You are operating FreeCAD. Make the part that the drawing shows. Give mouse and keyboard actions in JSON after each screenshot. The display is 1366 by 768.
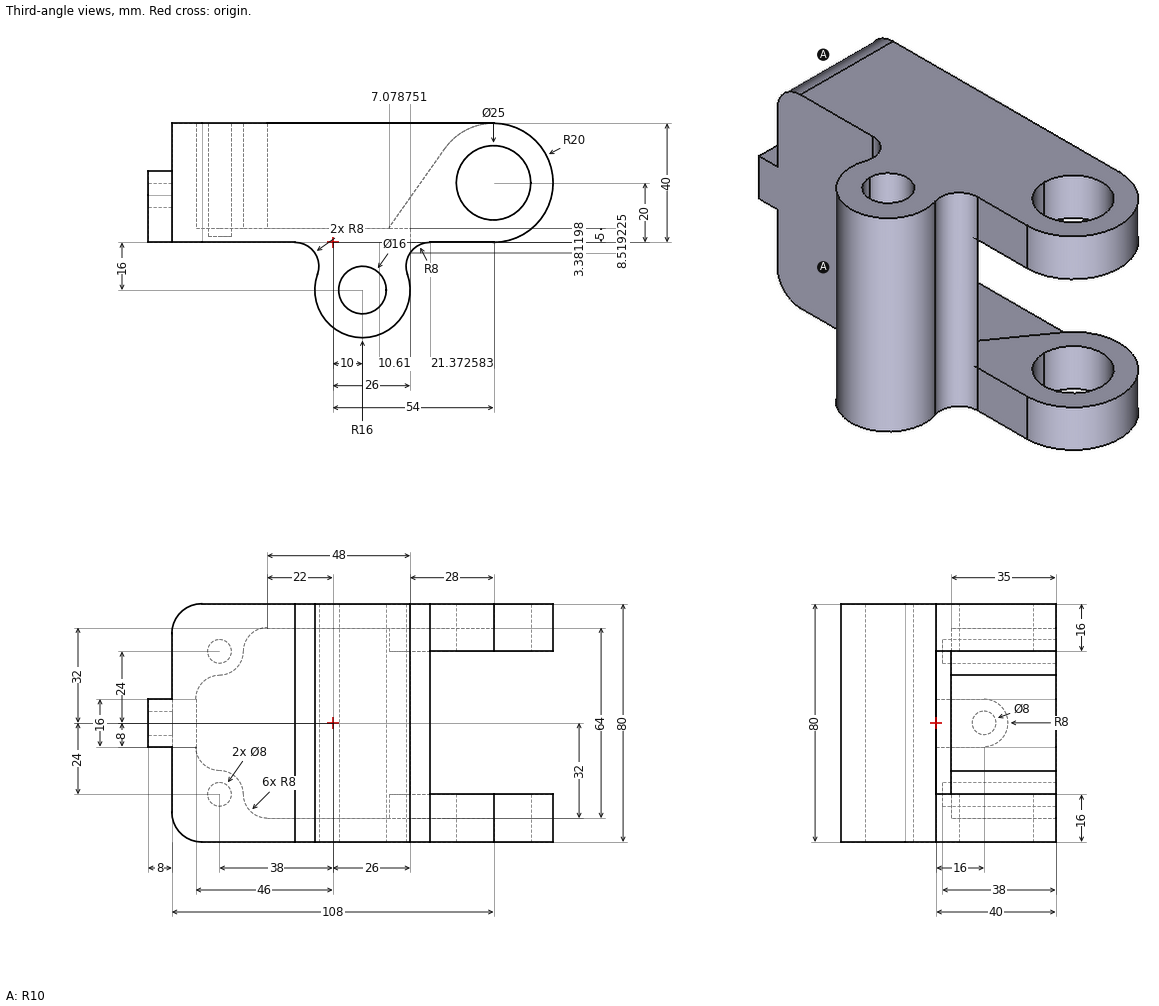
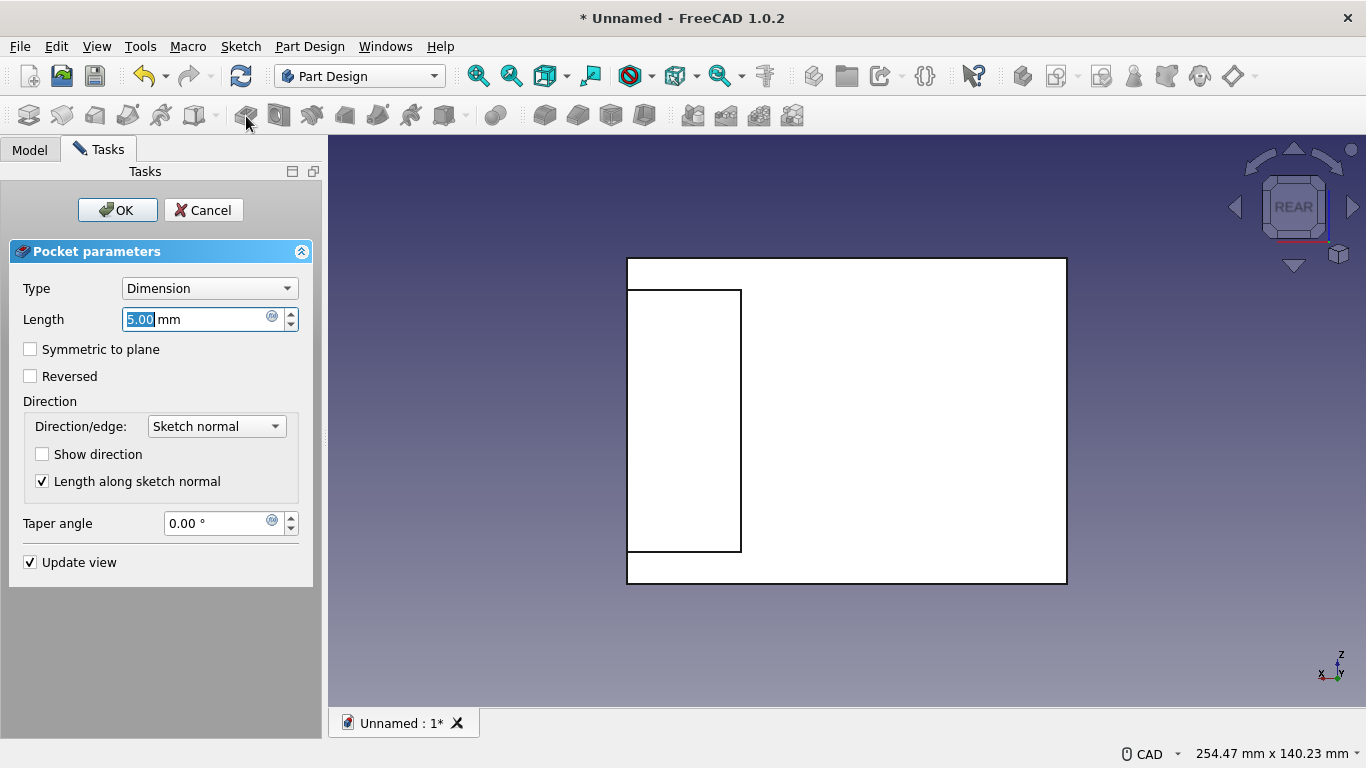
{"action": "type", "text": "40"}
{"action": "key", "text": "Tab"}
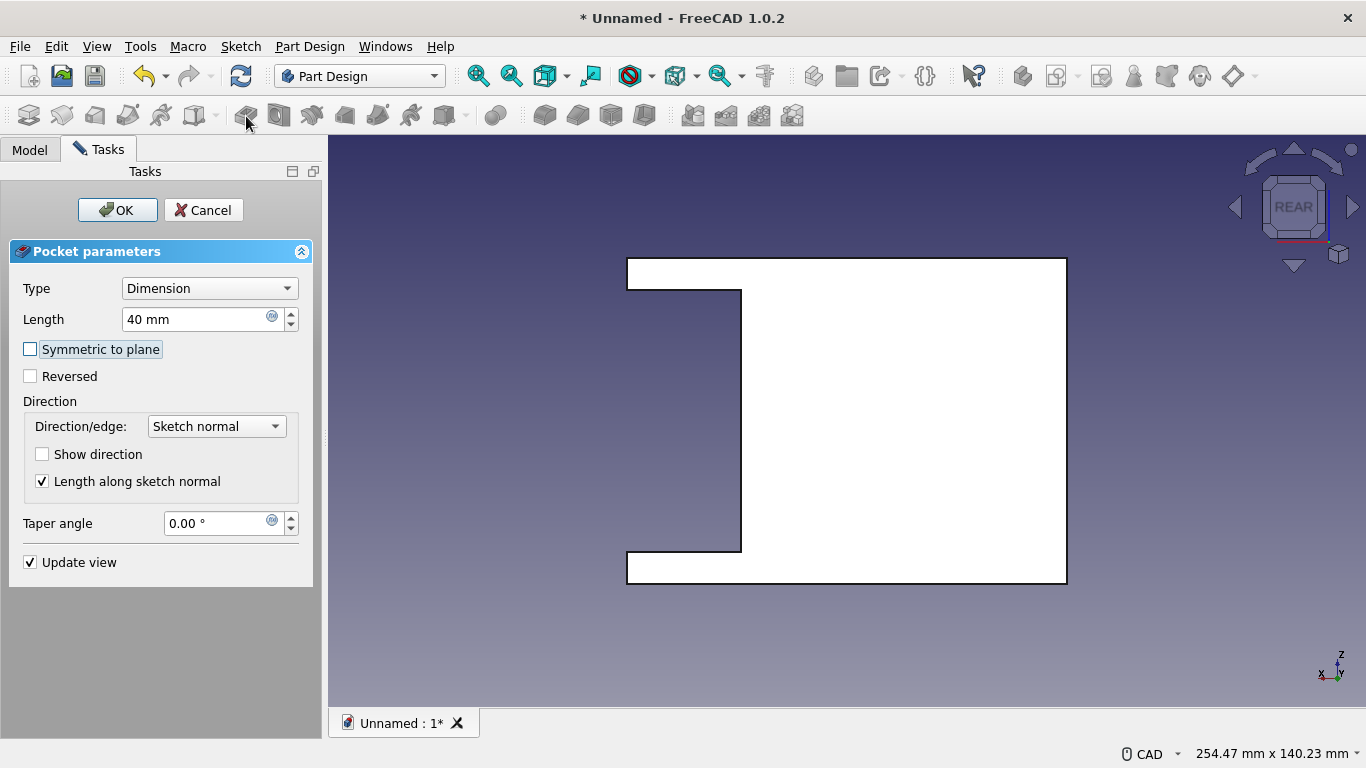
{"action": "left_click", "coordinate": [118, 210]}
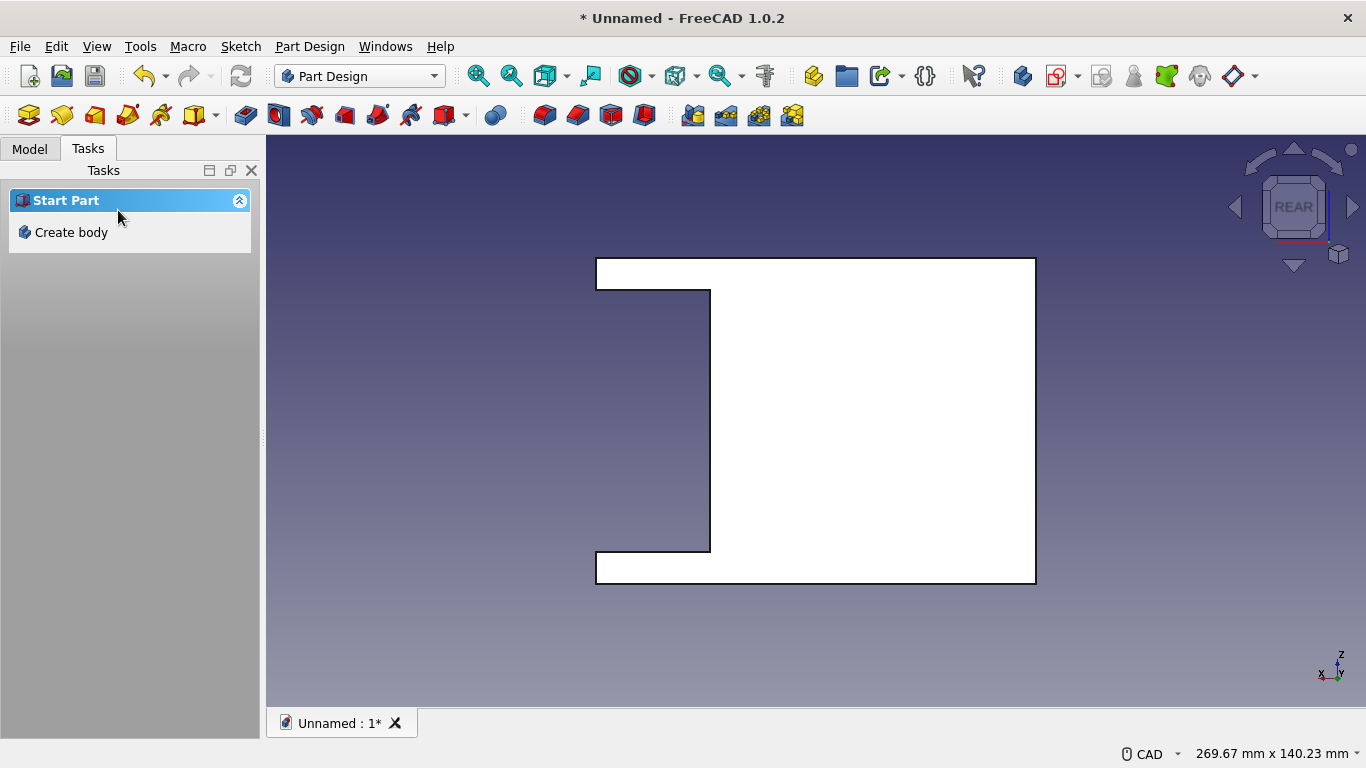
{"action": "left_click", "coordinate": [879, 420]}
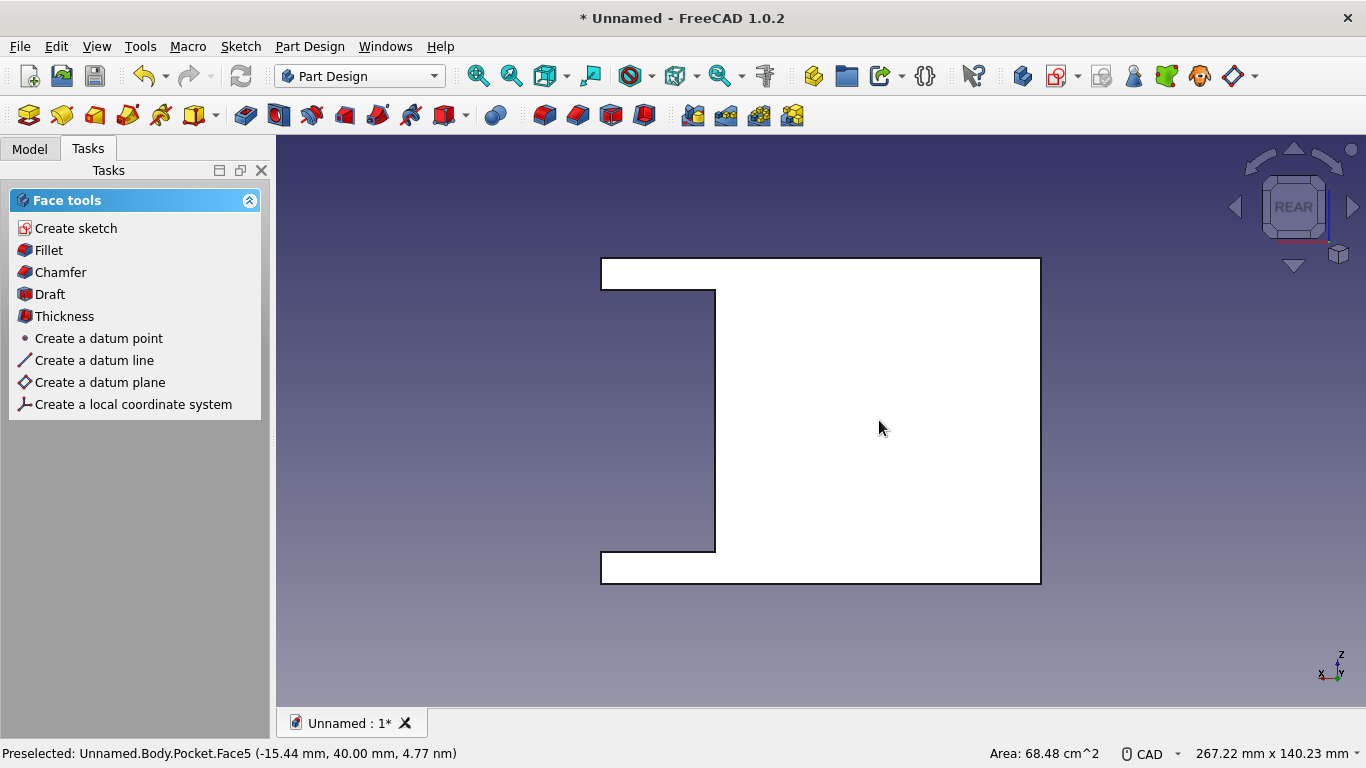
{"action": "left_click", "coordinate": [1056, 76]}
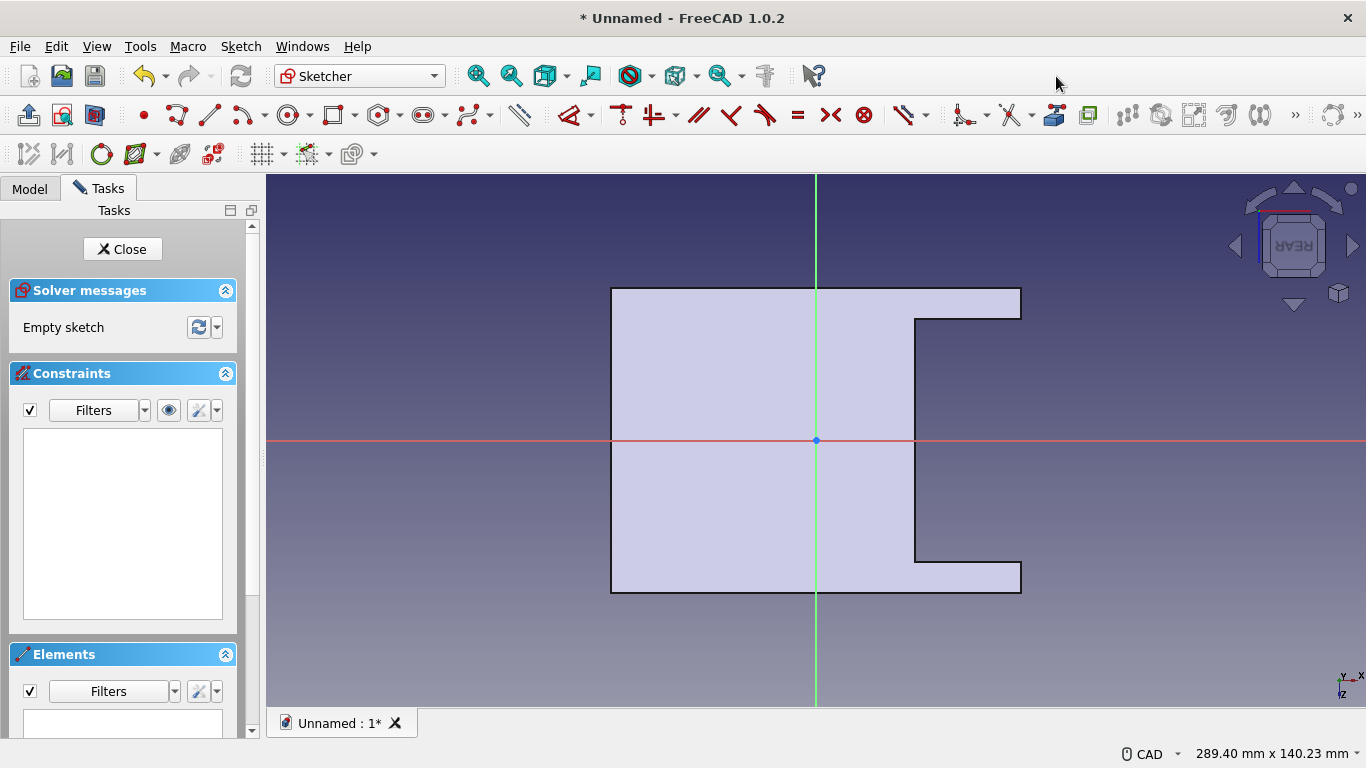
{"action": "scroll", "coordinate": [840, 440], "scroll_direction": "up", "scroll_amount": 2}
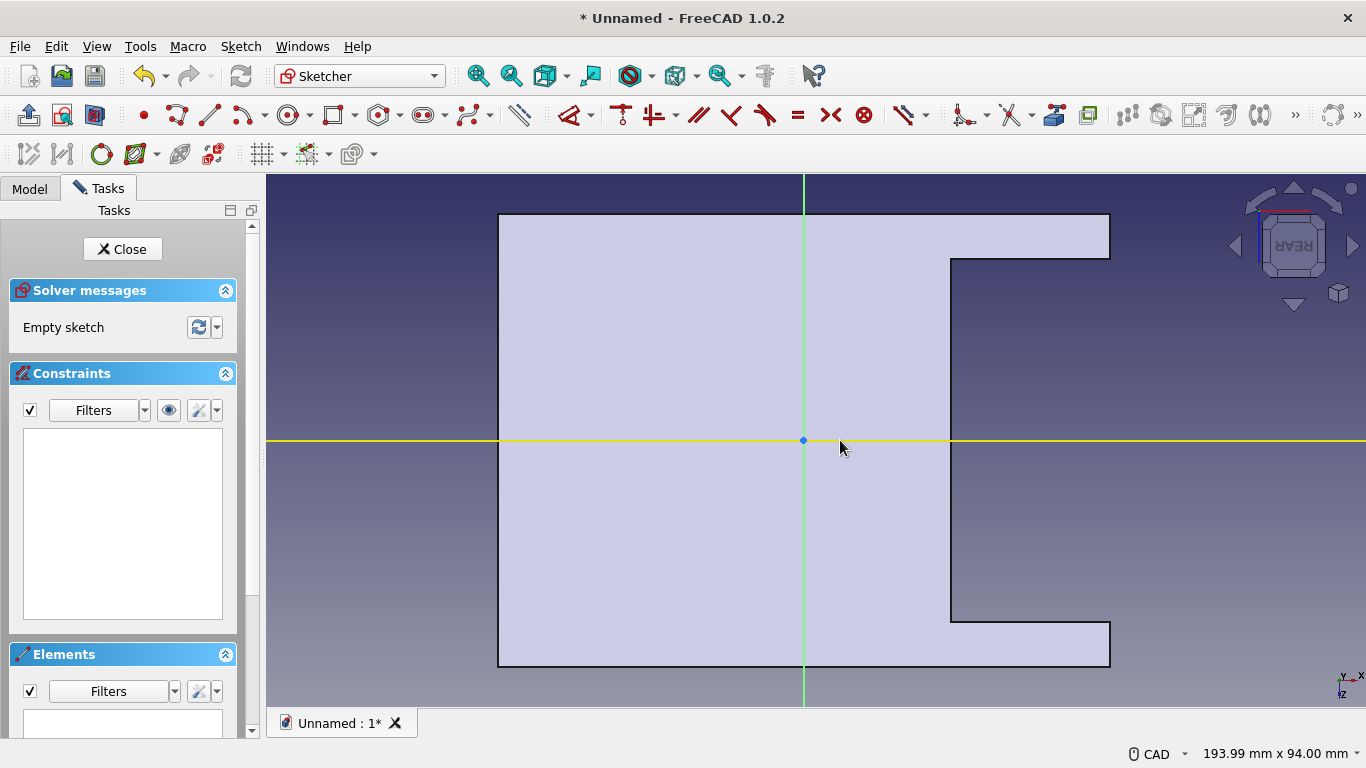
{"action": "key", "text": "g m"}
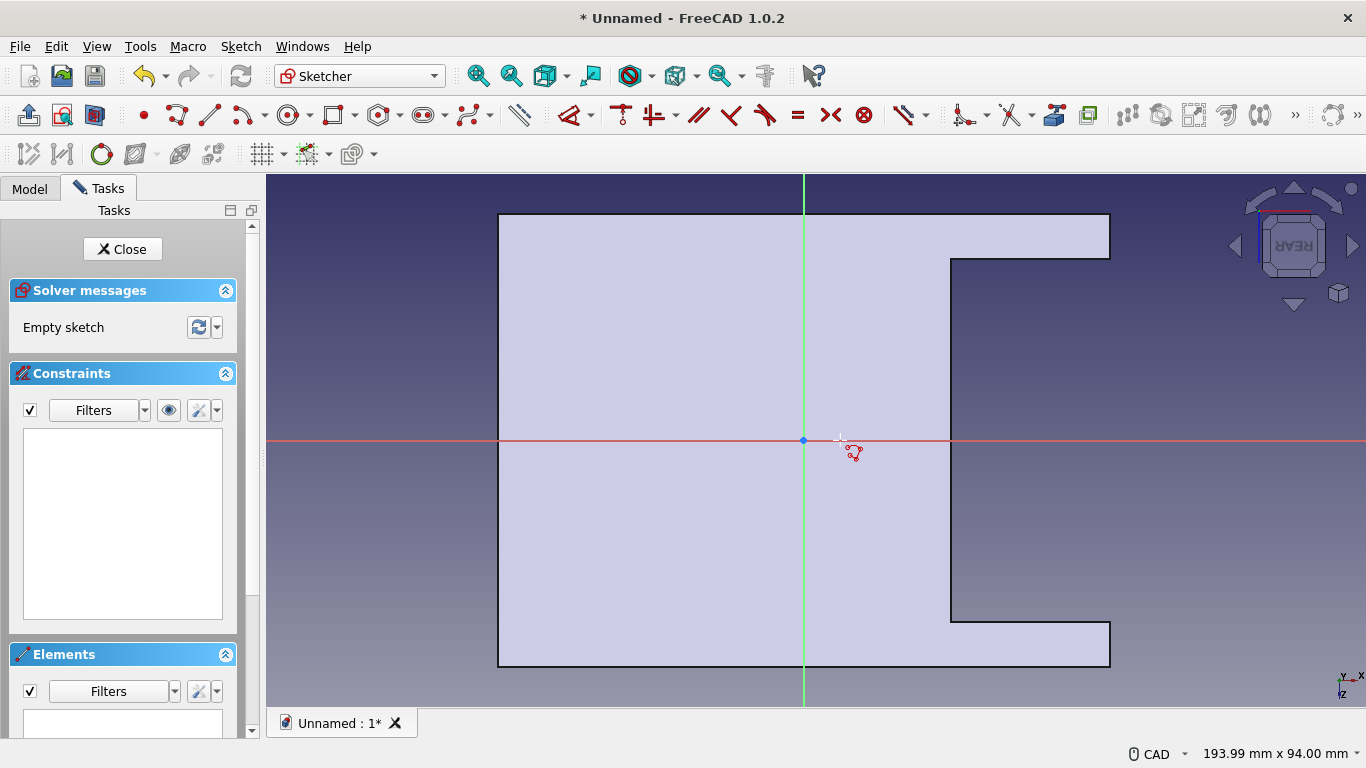
{"action": "left_click", "coordinate": [679, 622]}
{"action": "left_click", "coordinate": [951, 622]}
{"action": "left_click", "coordinate": [951, 259]}
{"action": "left_click", "coordinate": [679, 259]}
{"action": "right_click", "coordinate": [679, 259]}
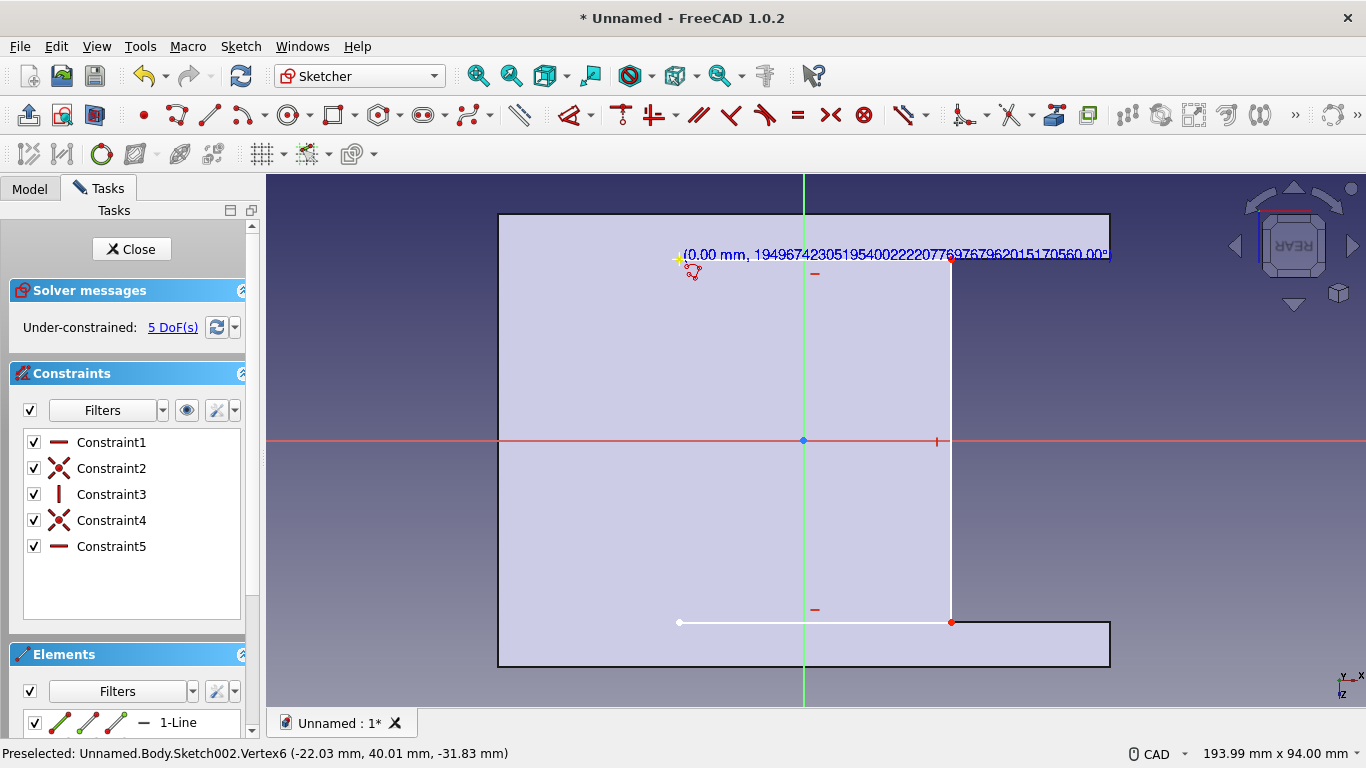
{"action": "left_click", "coordinate": [210, 116]}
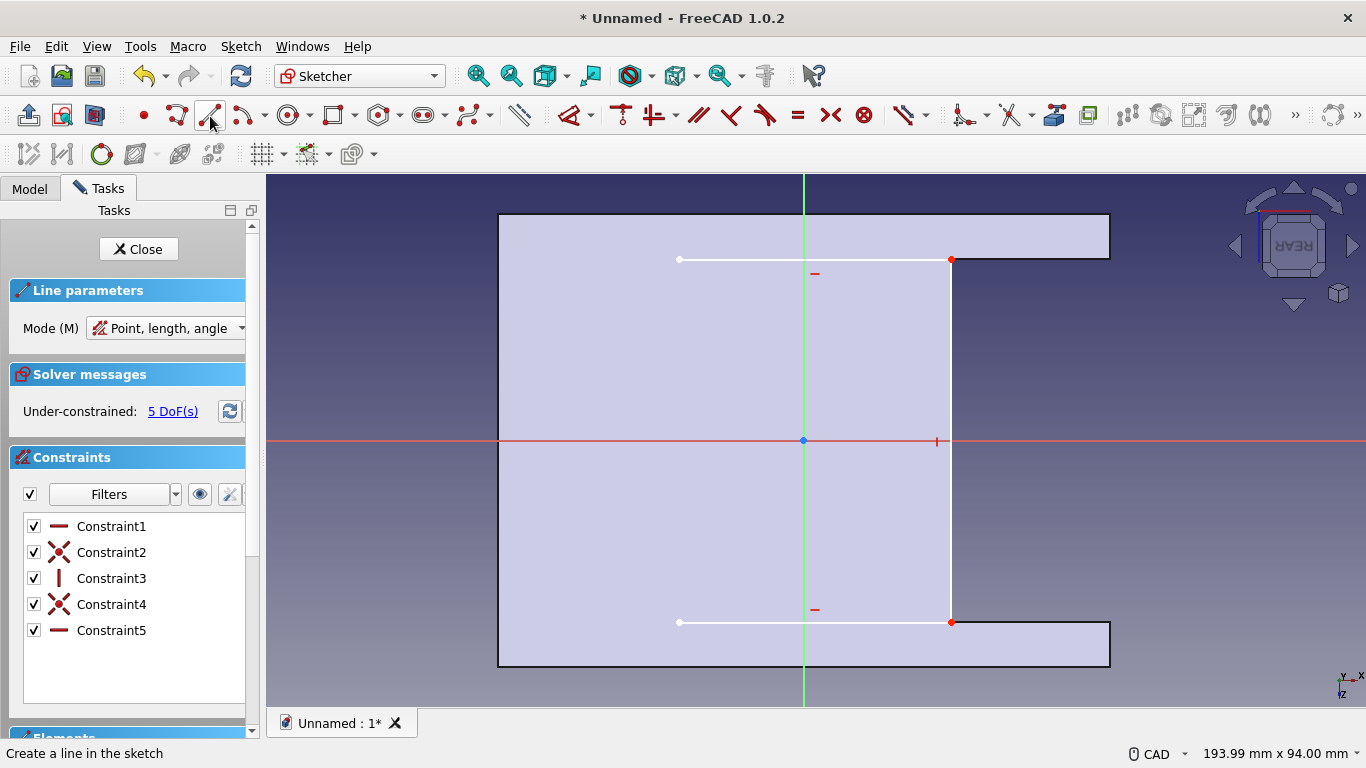
{"action": "left_click", "coordinate": [543, 395]}
{"action": "left_click", "coordinate": [543, 486]}